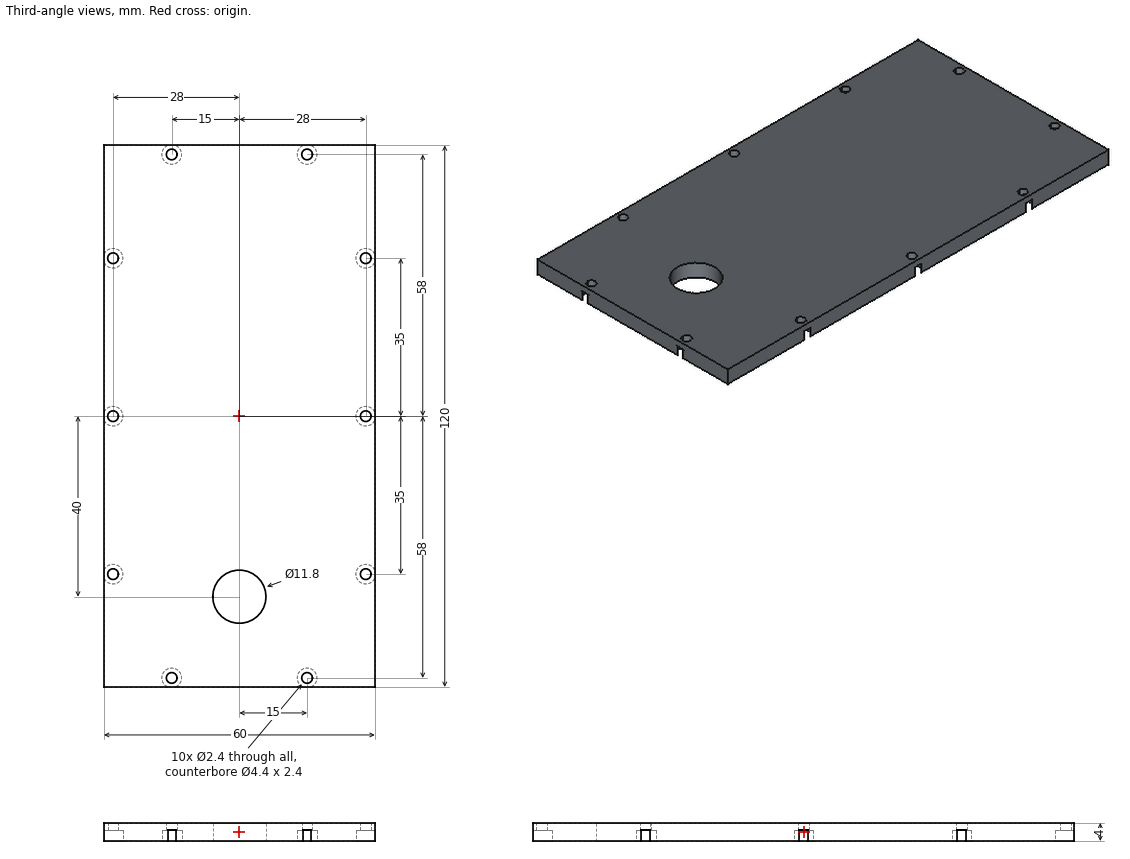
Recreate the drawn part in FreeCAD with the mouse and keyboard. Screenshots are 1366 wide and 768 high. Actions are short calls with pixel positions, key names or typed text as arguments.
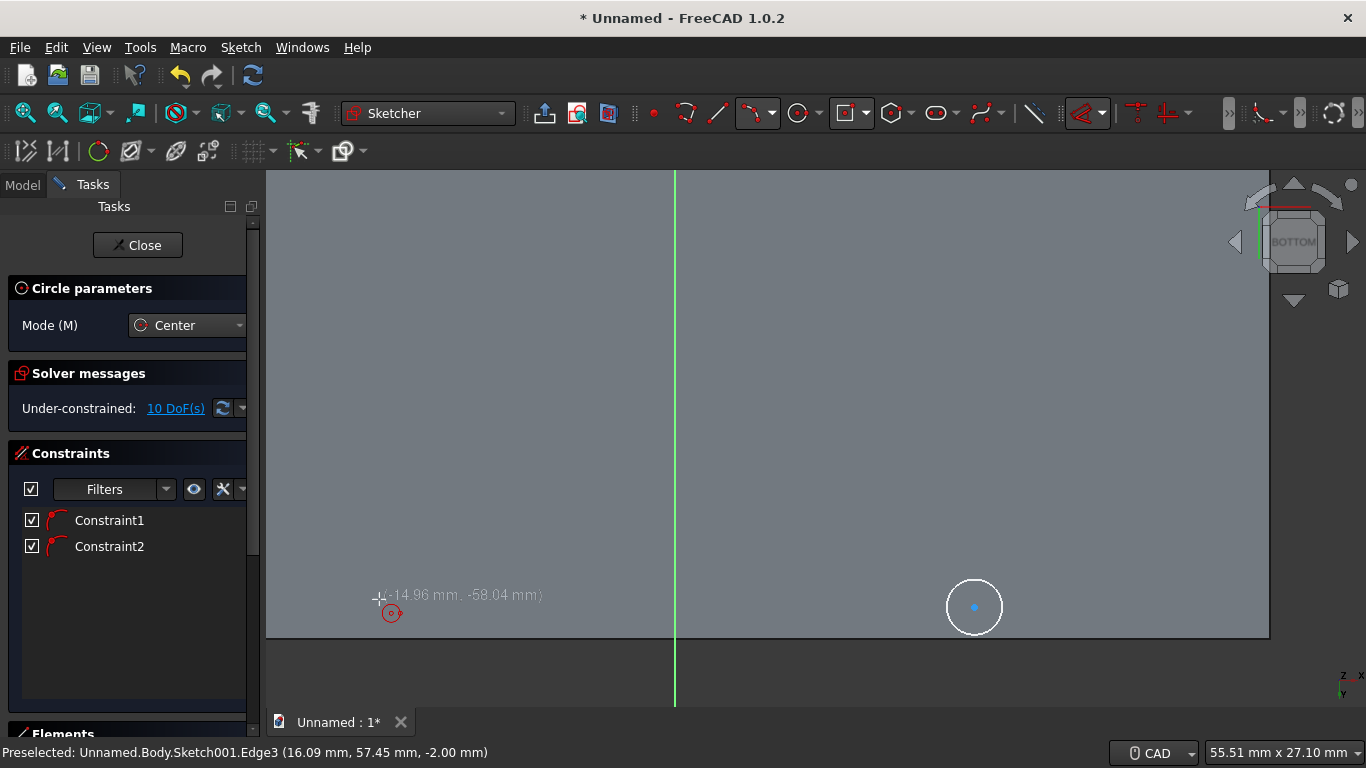
scroll(759, 593, down, 10)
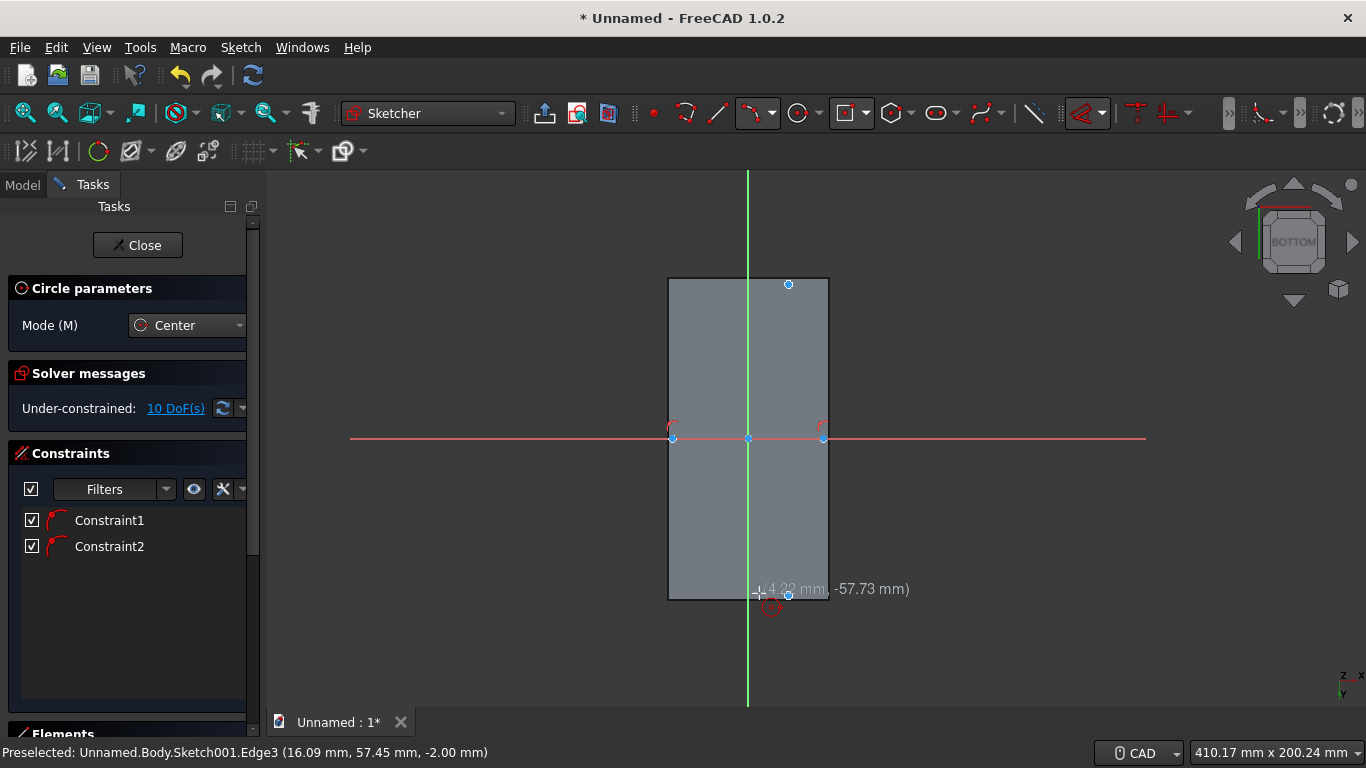
click(708, 595)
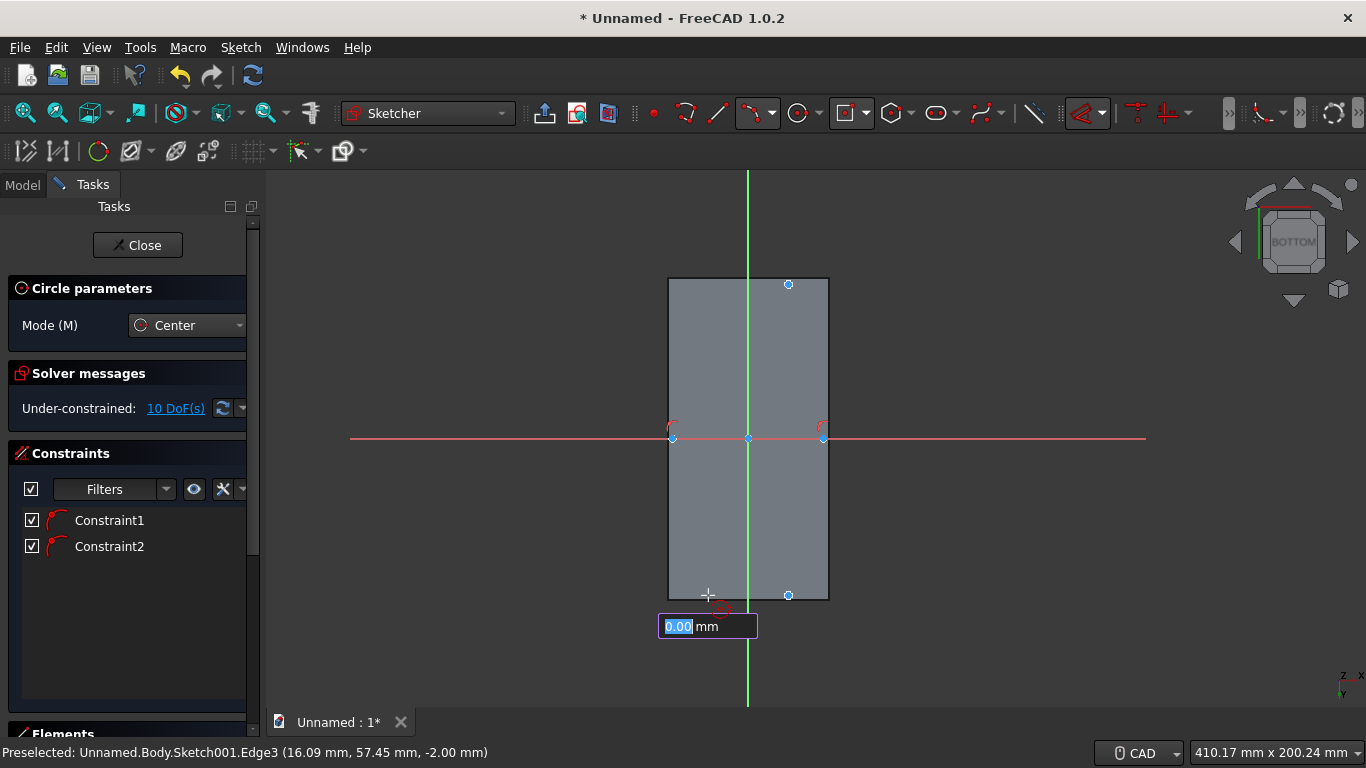
scroll(710, 592, up, 8)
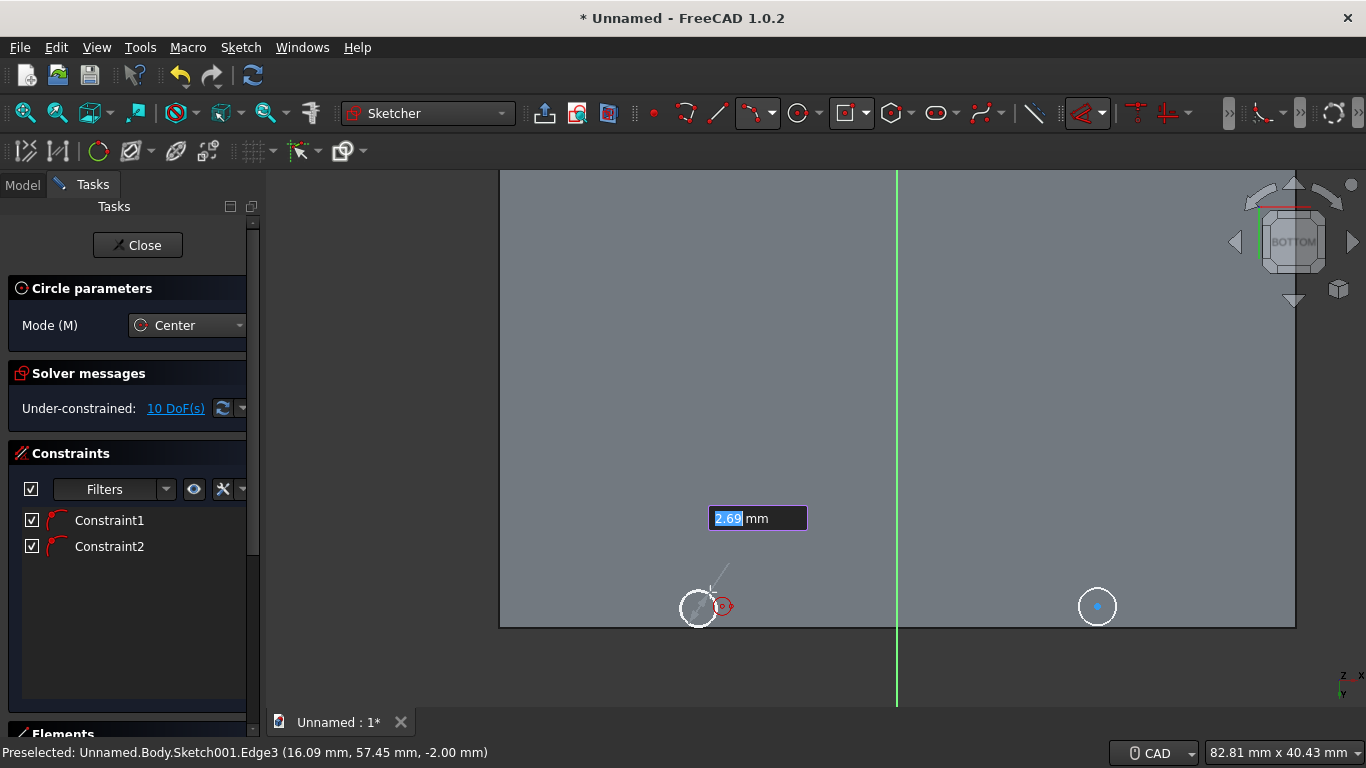
click(709, 590)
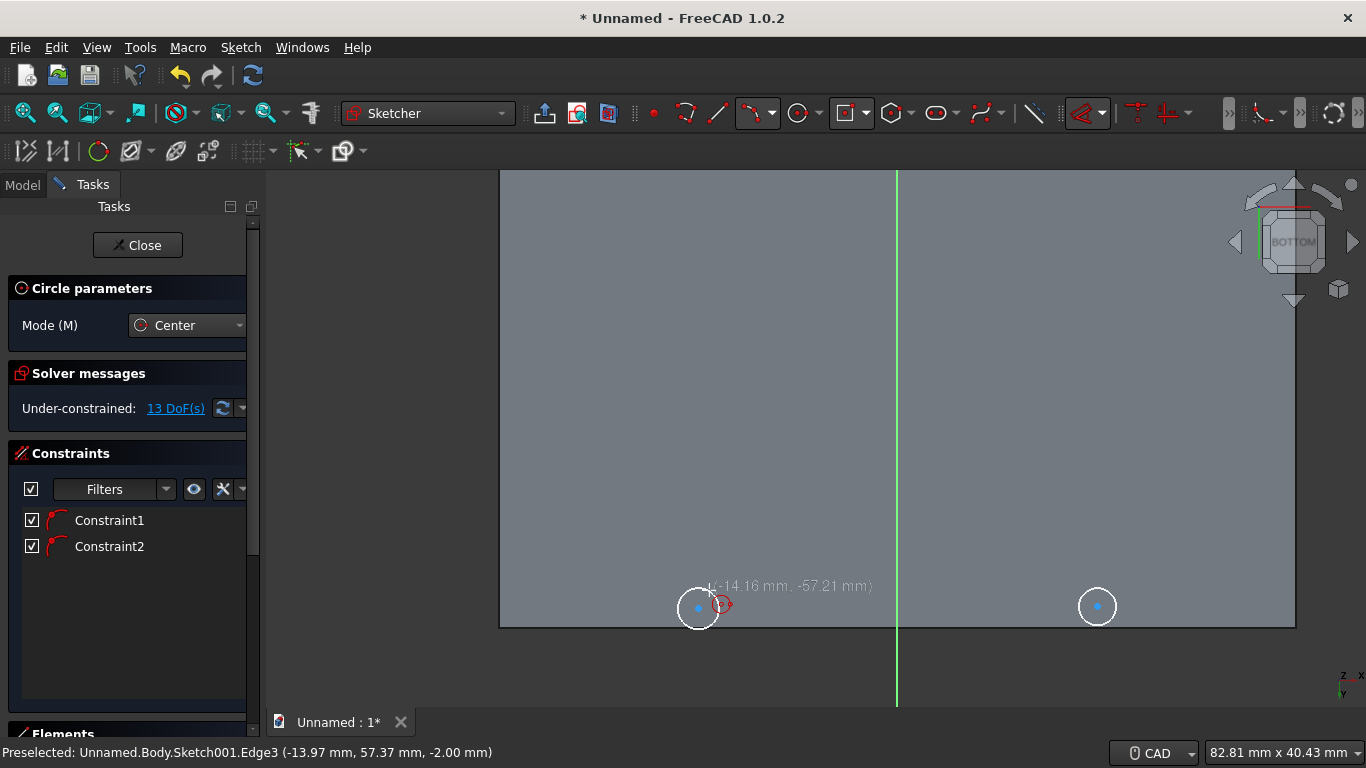
scroll(710, 592, down, 8)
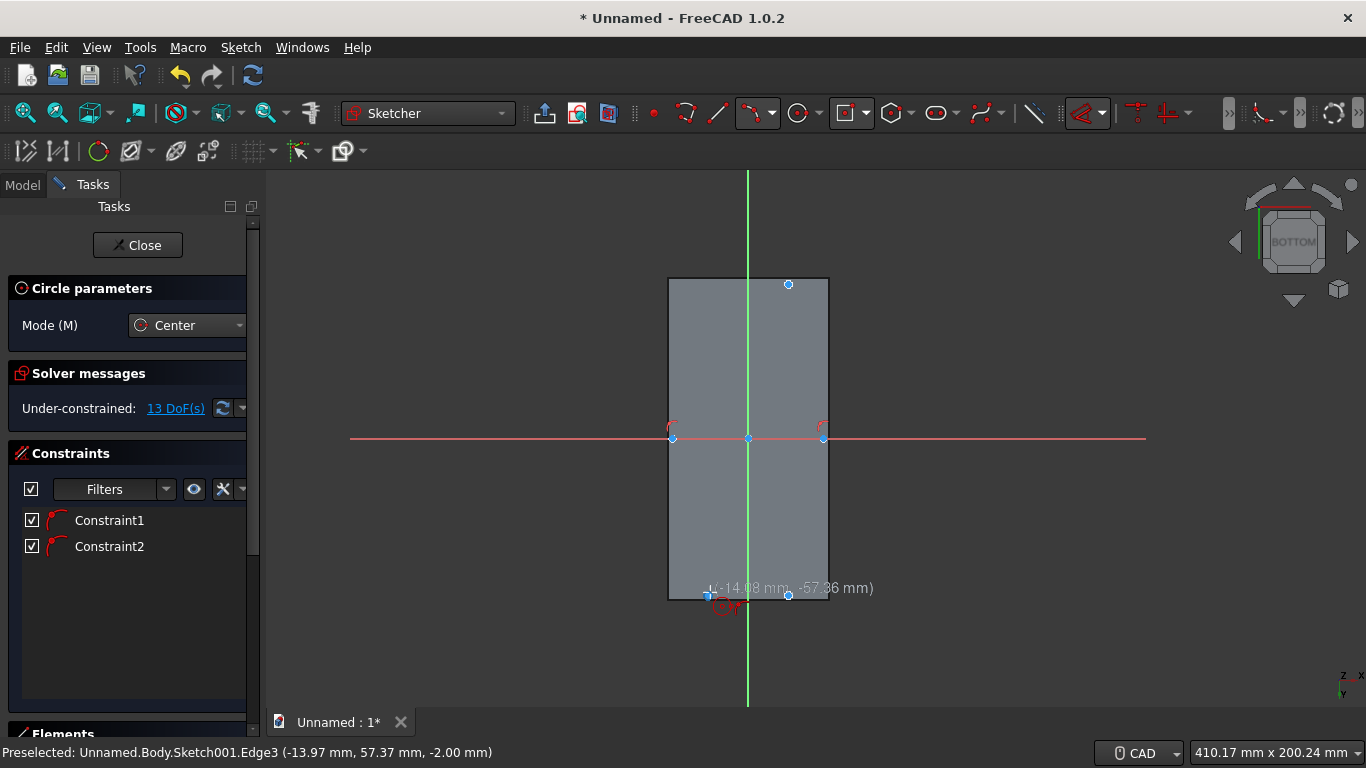
scroll(823, 533, up, 10)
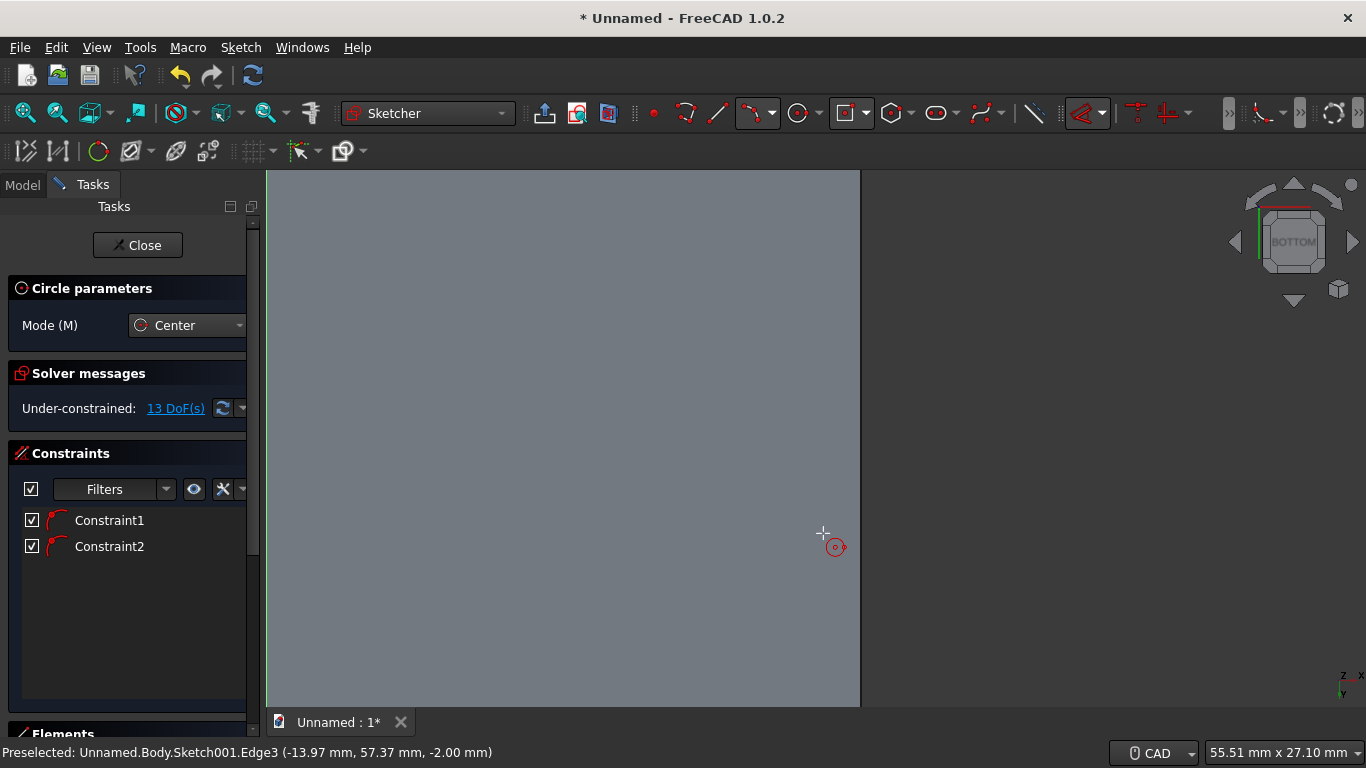
scroll(823, 533, down, 10)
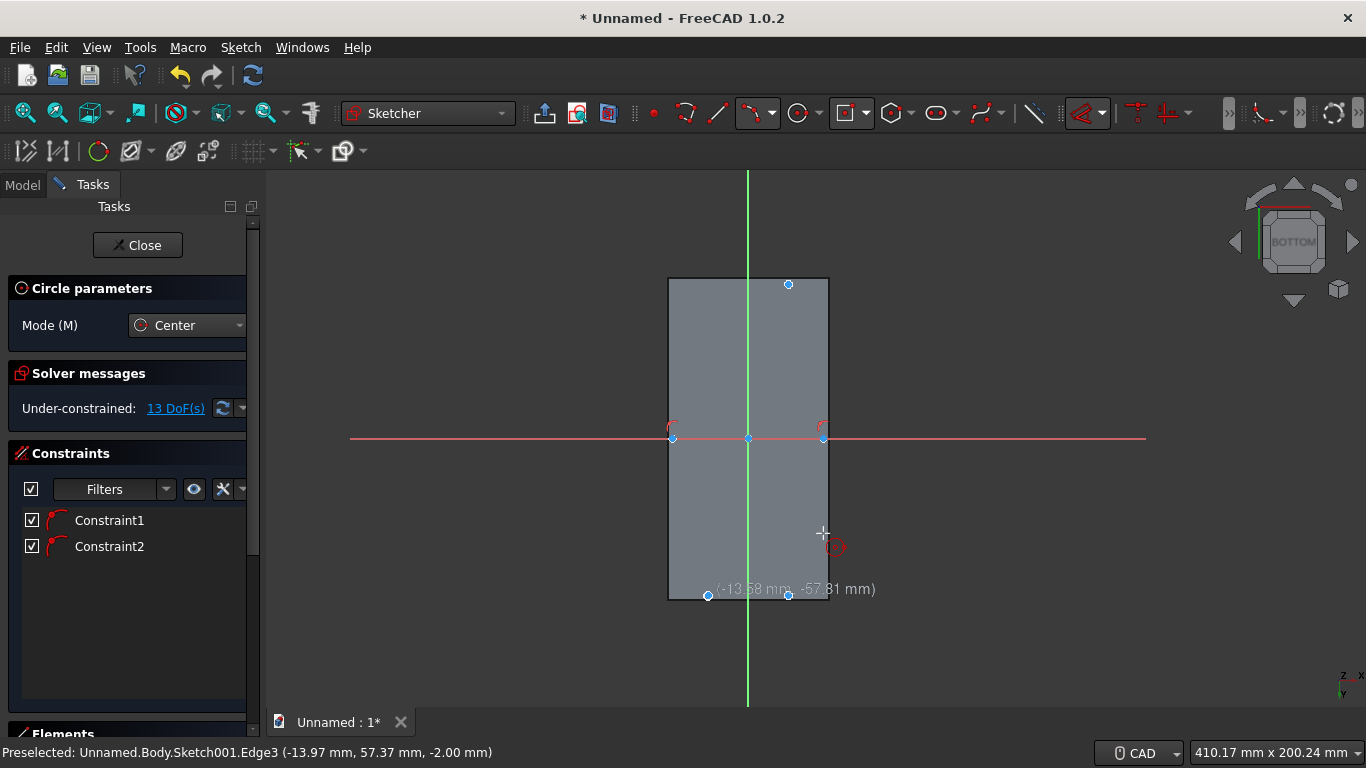
click(823, 533)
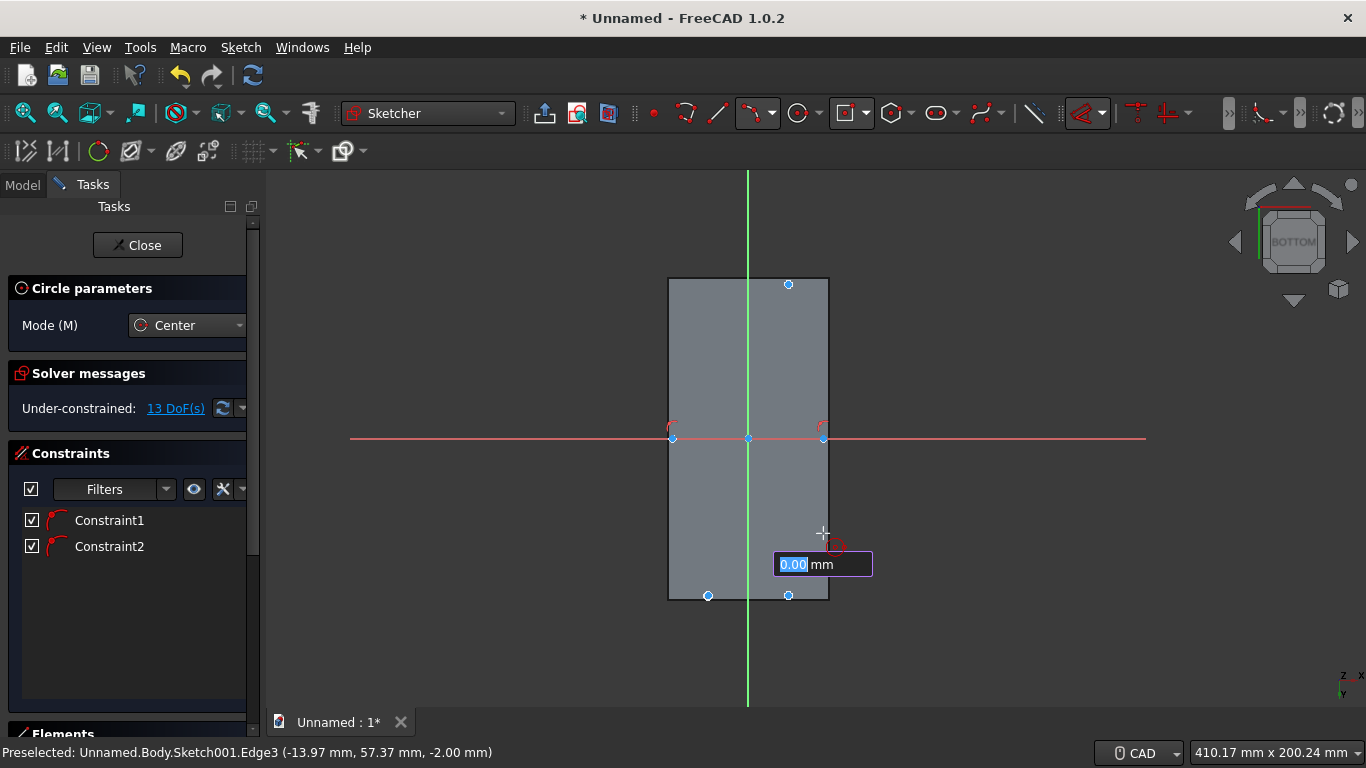
scroll(825, 531, up, 8)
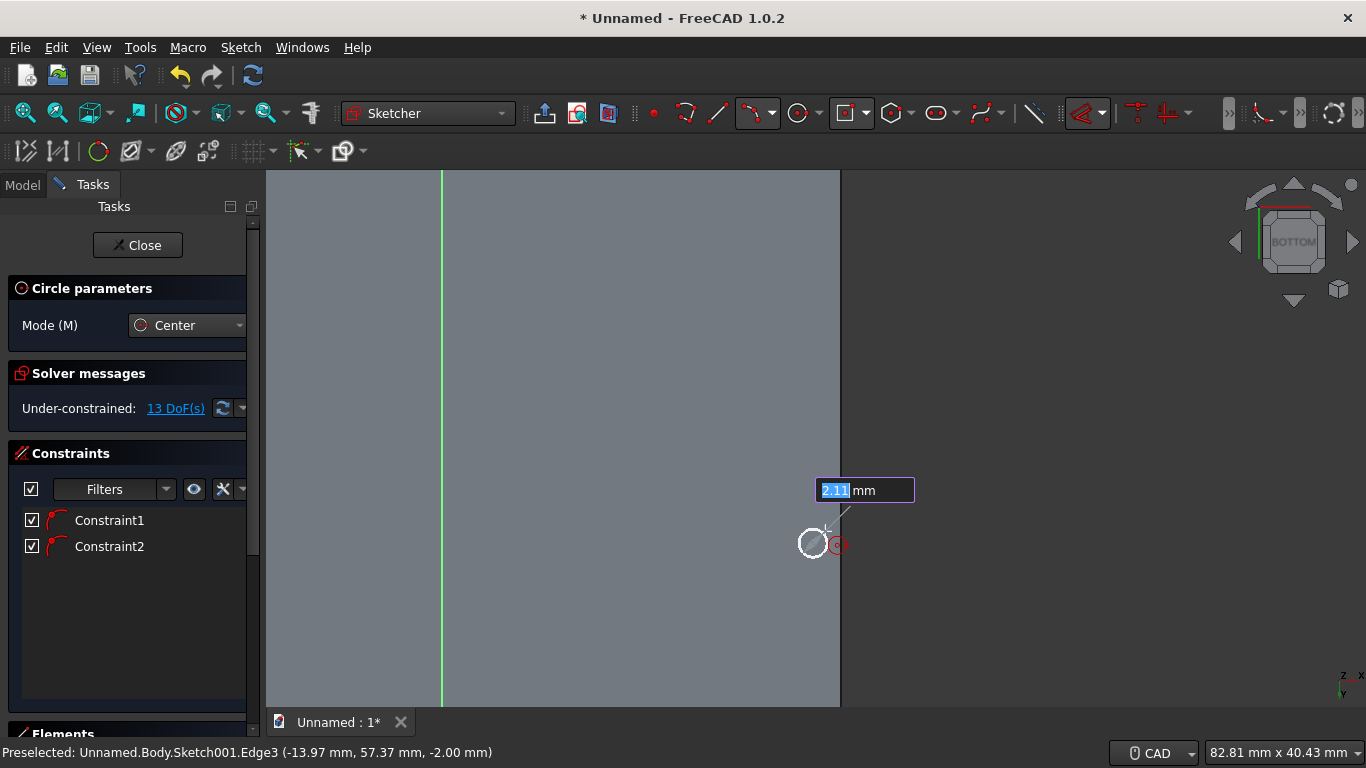
click(825, 526)